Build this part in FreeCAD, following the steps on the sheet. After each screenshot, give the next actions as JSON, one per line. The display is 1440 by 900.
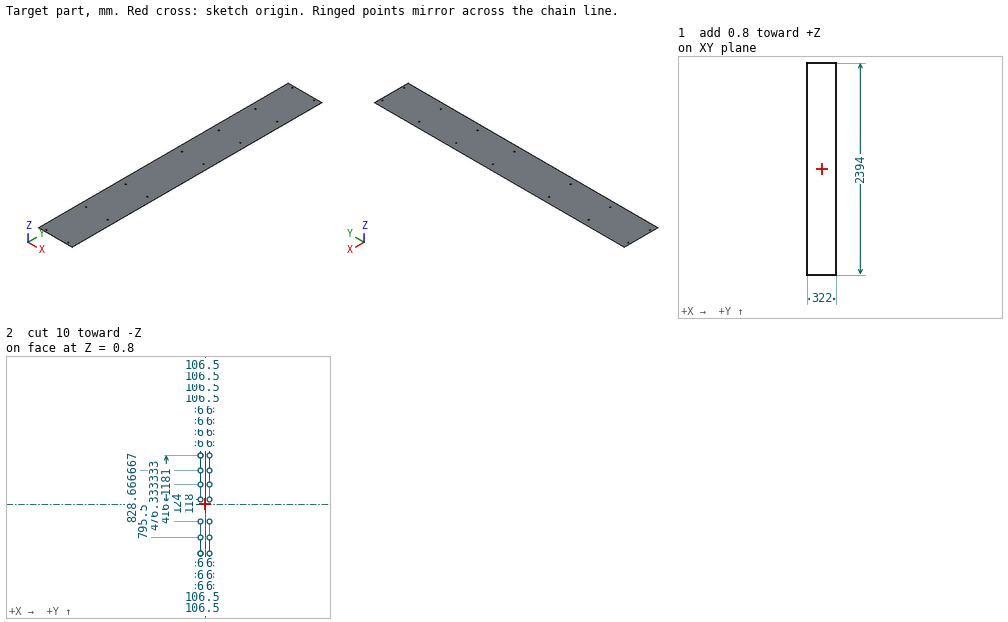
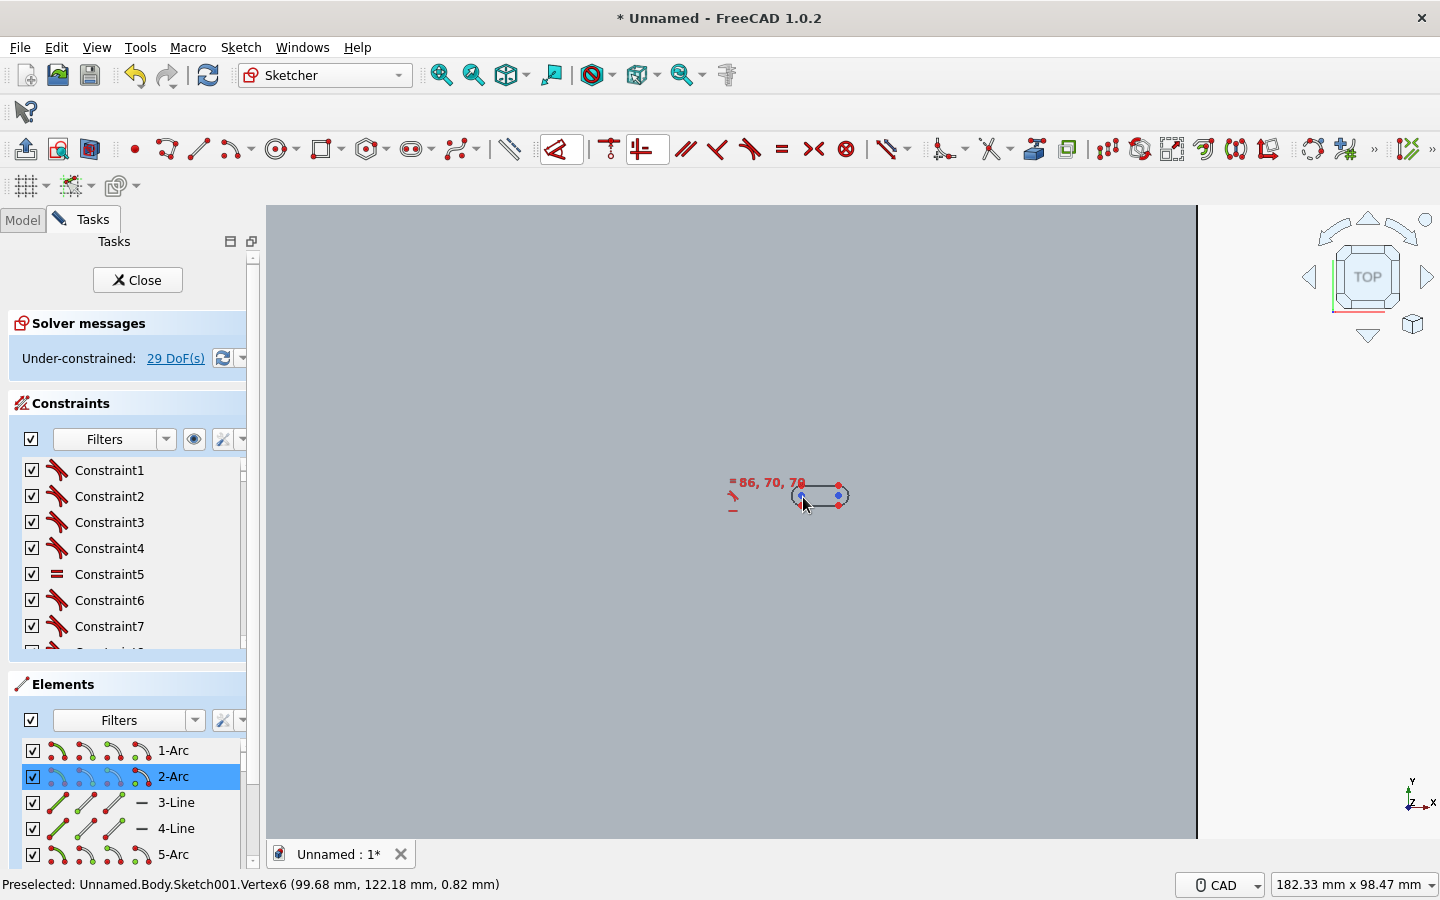
{"action": "scroll", "coordinate": [802, 496], "scroll_direction": "up", "scroll_amount": 4}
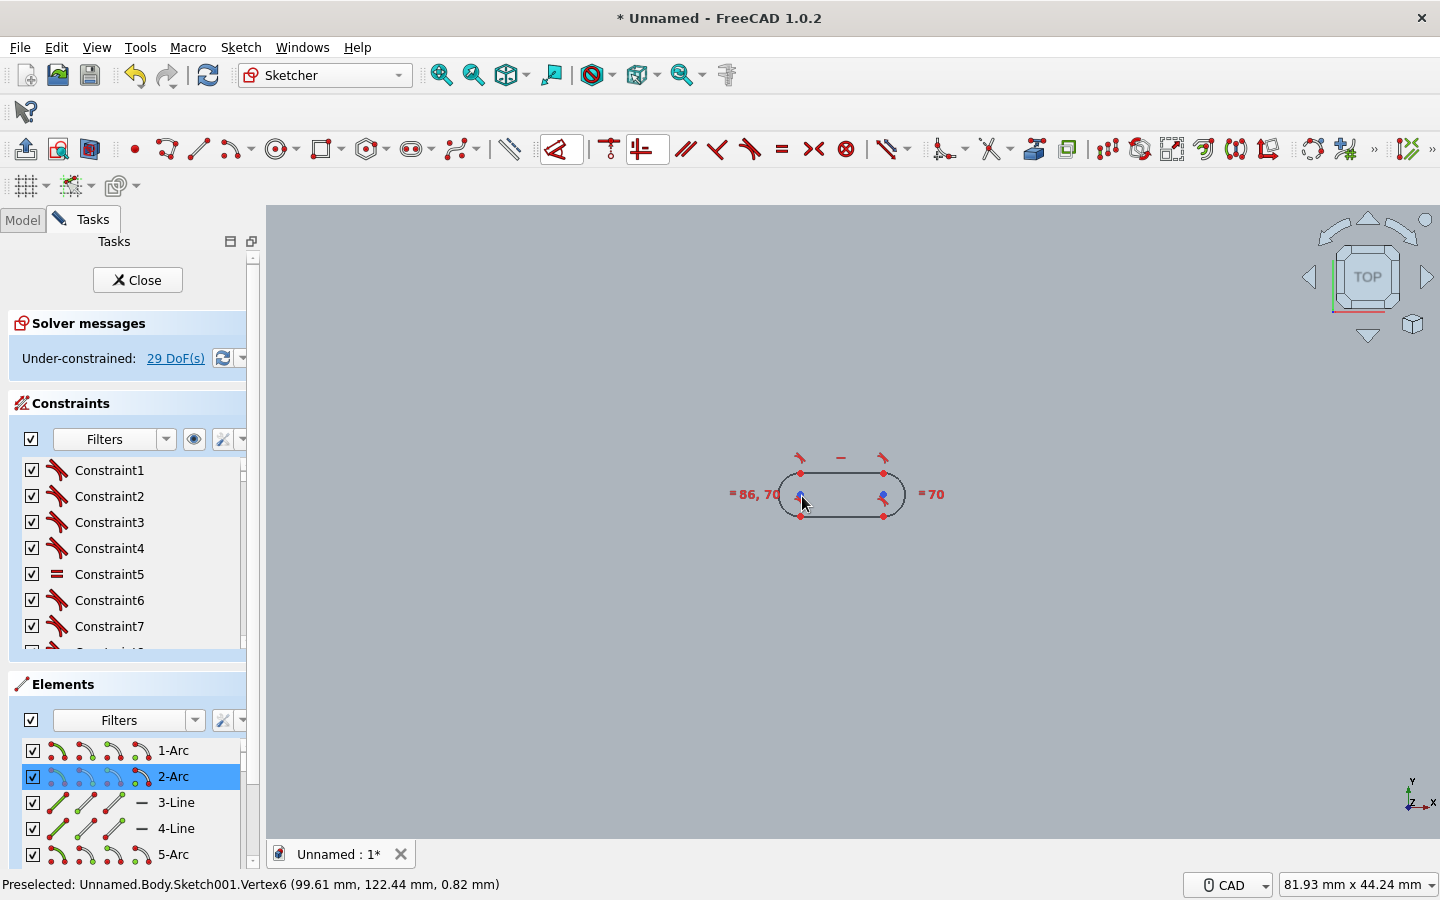
{"action": "left_click", "coordinate": [800, 495]}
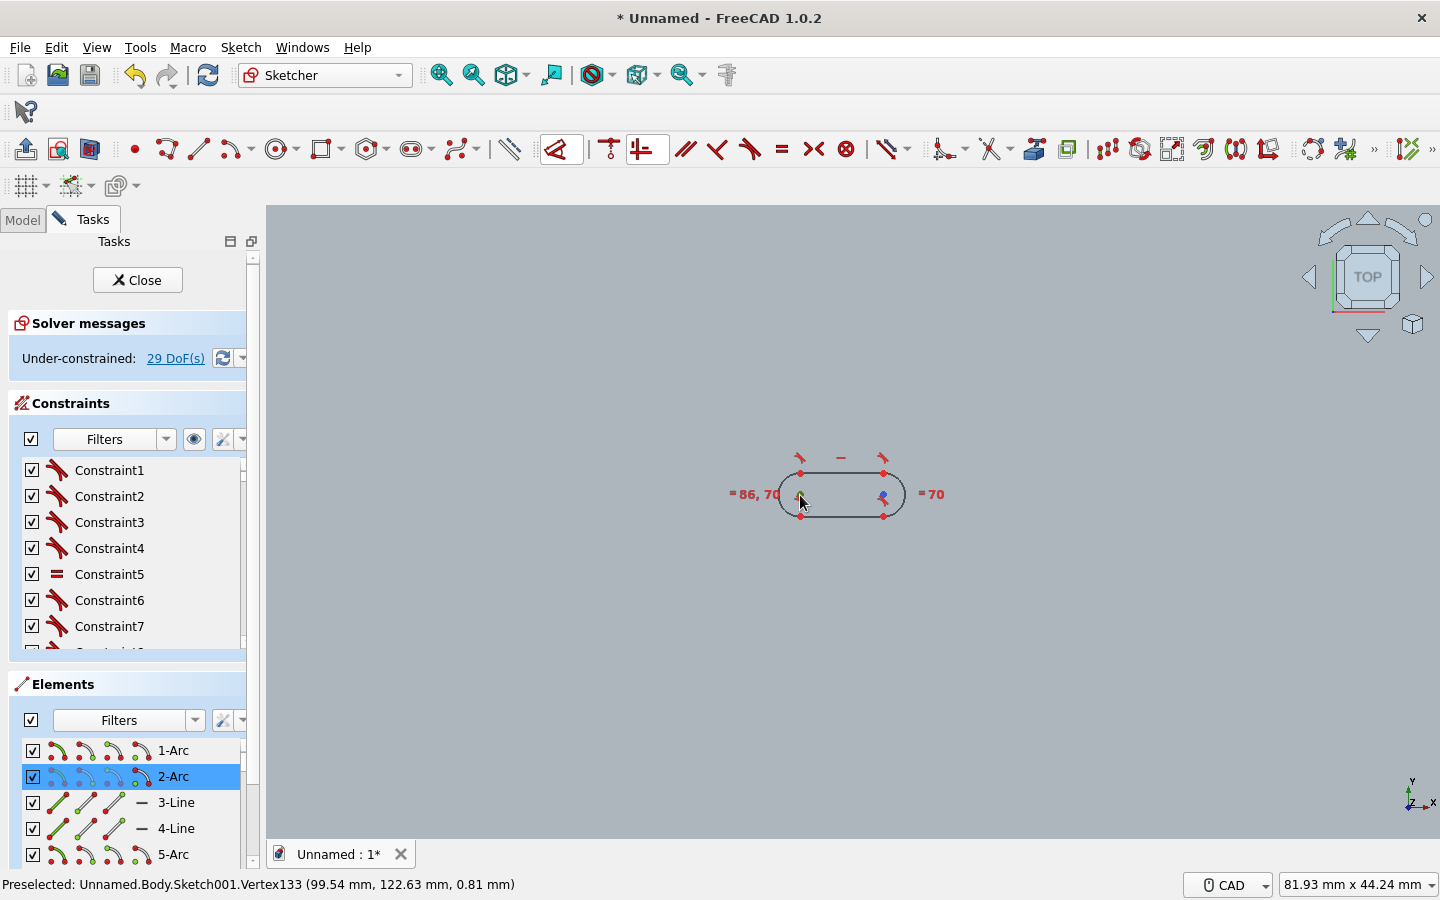
{"action": "scroll", "coordinate": [784, 522], "scroll_direction": "down", "scroll_amount": 15}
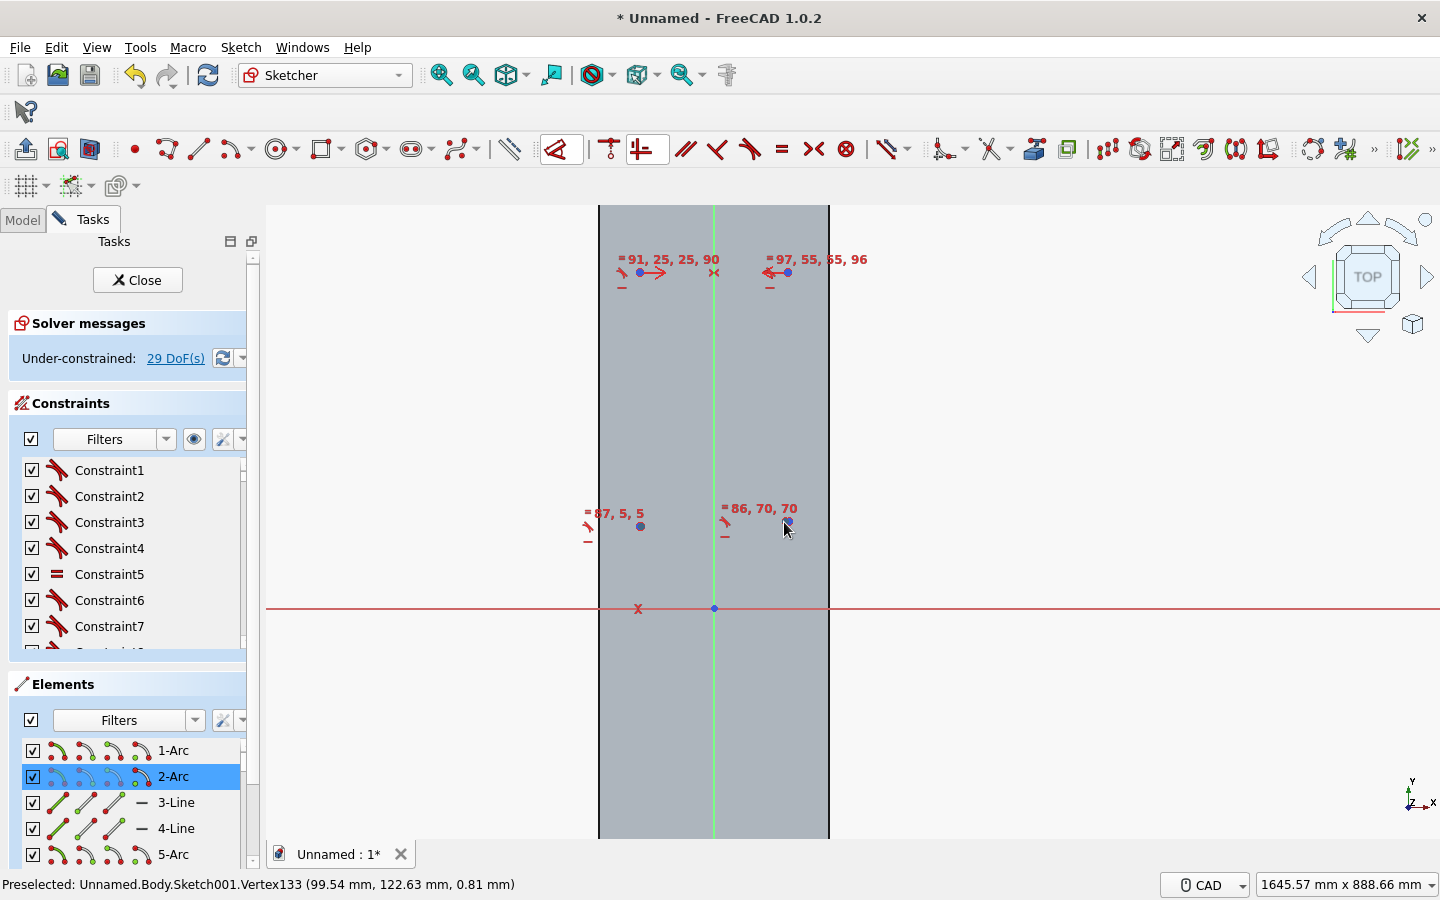
{"action": "scroll", "coordinate": [808, 494], "scroll_direction": "down", "scroll_amount": 7}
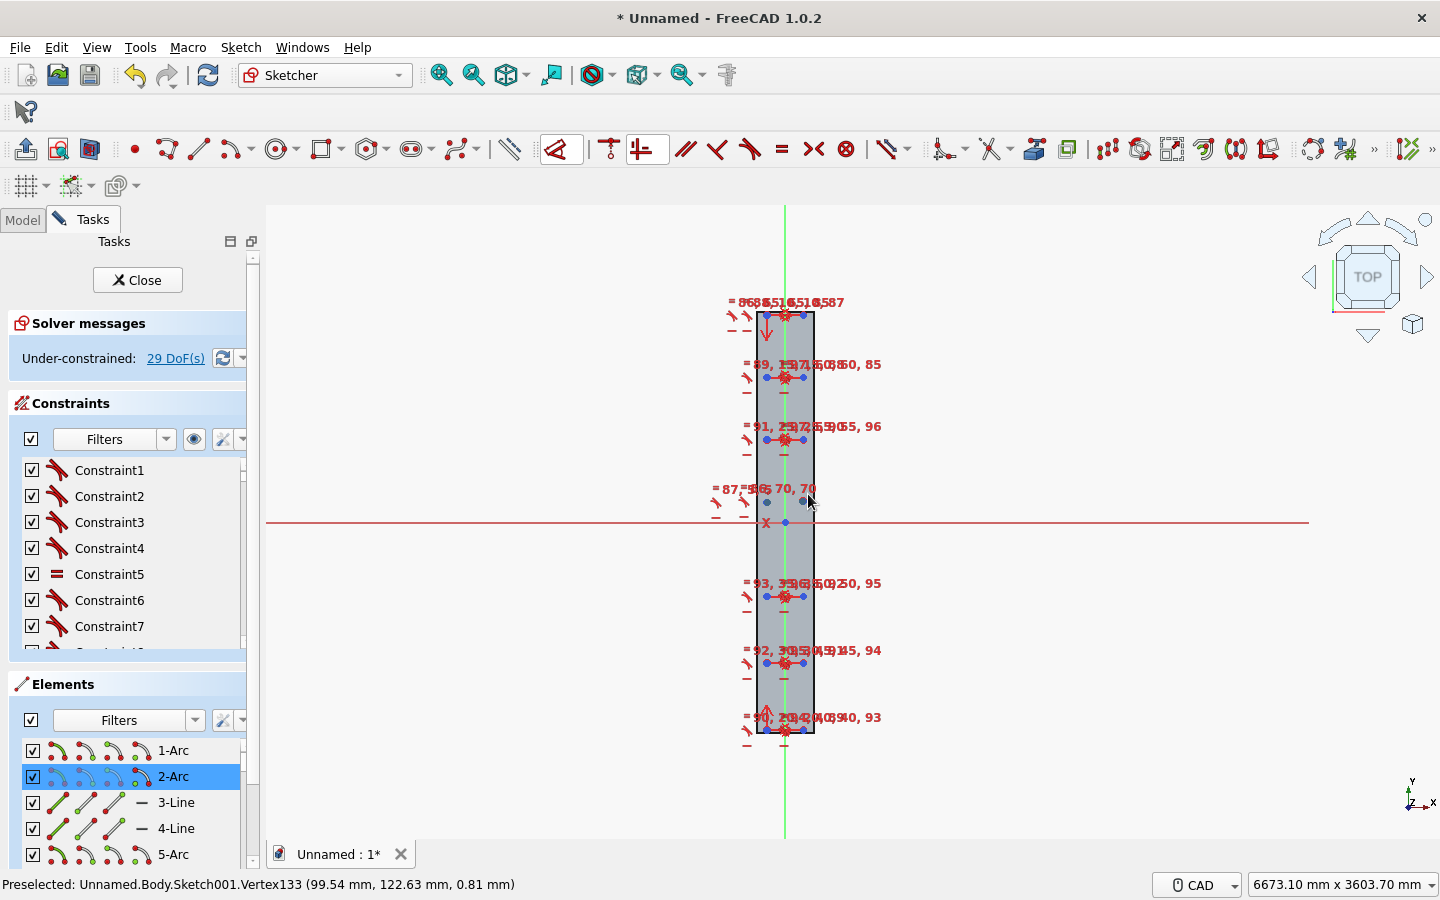
{"action": "left_click", "coordinate": [785, 770]}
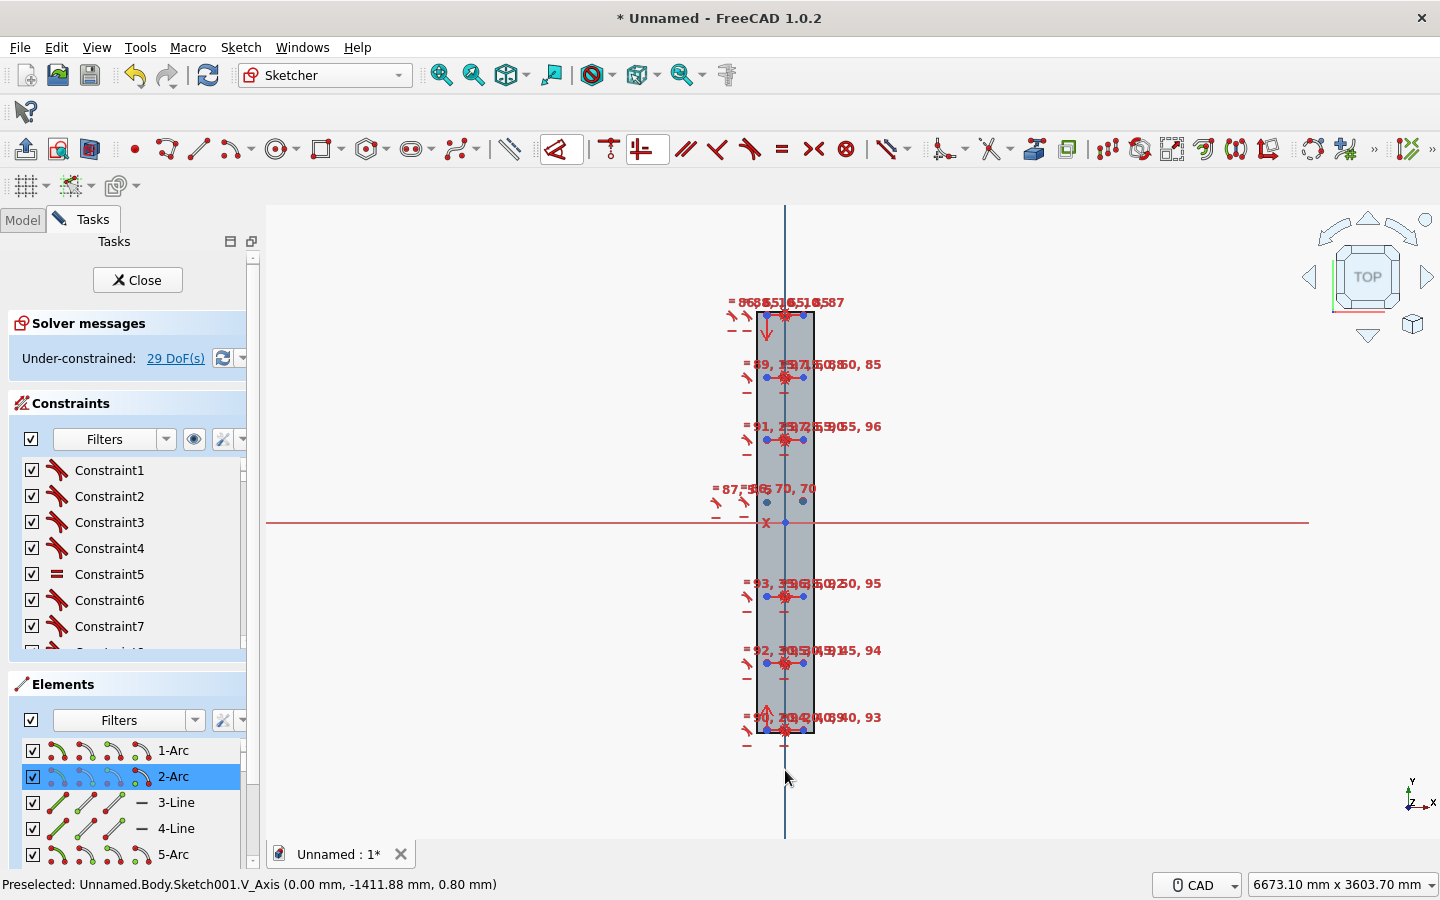
{"action": "left_click", "coordinate": [814, 150]}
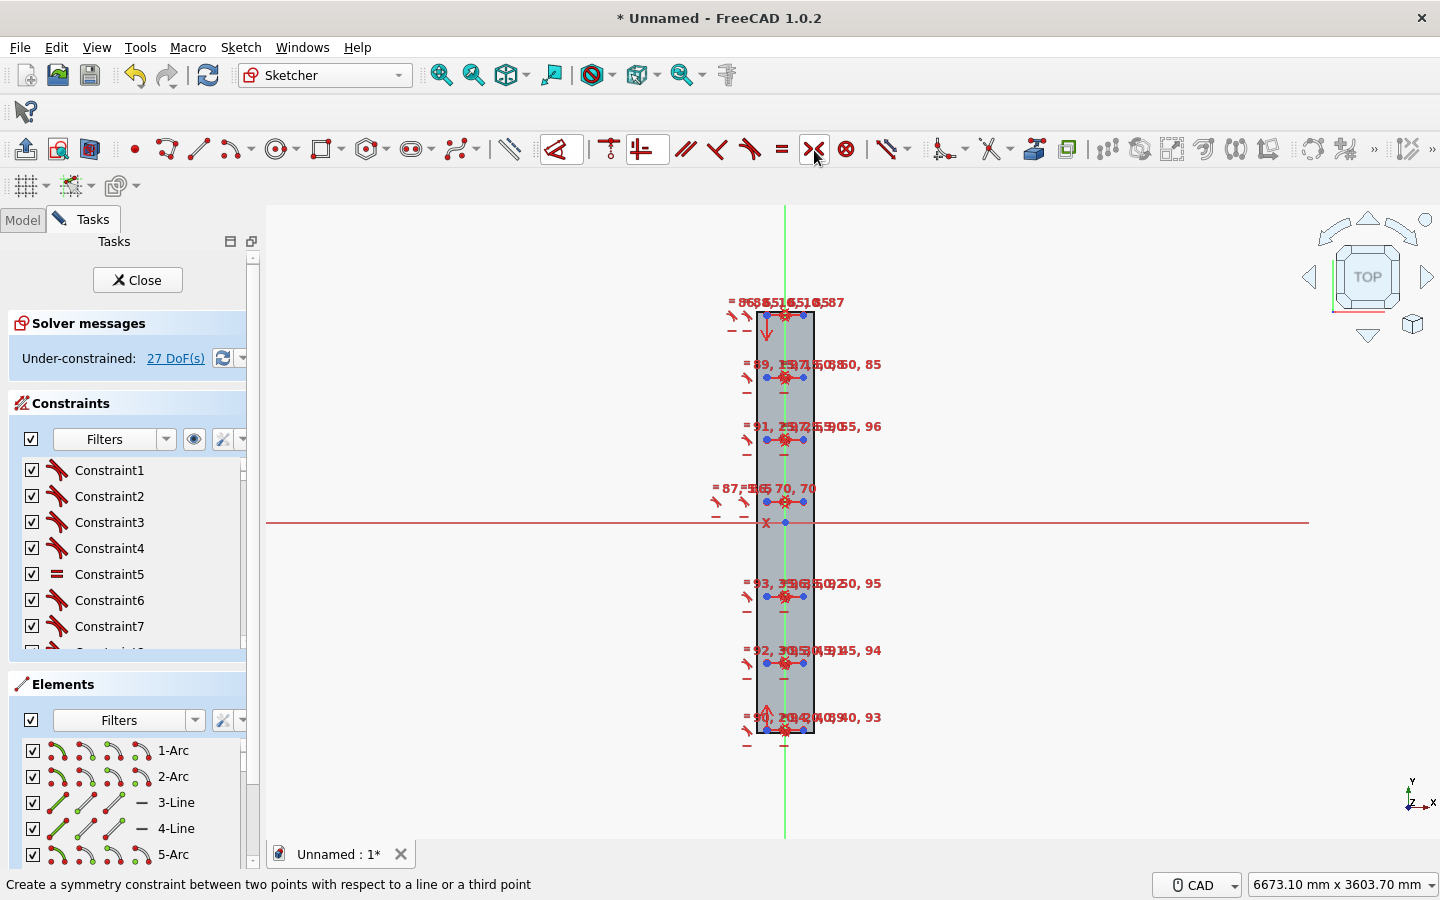
{"action": "scroll", "coordinate": [767, 502], "scroll_direction": "up", "scroll_amount": 19}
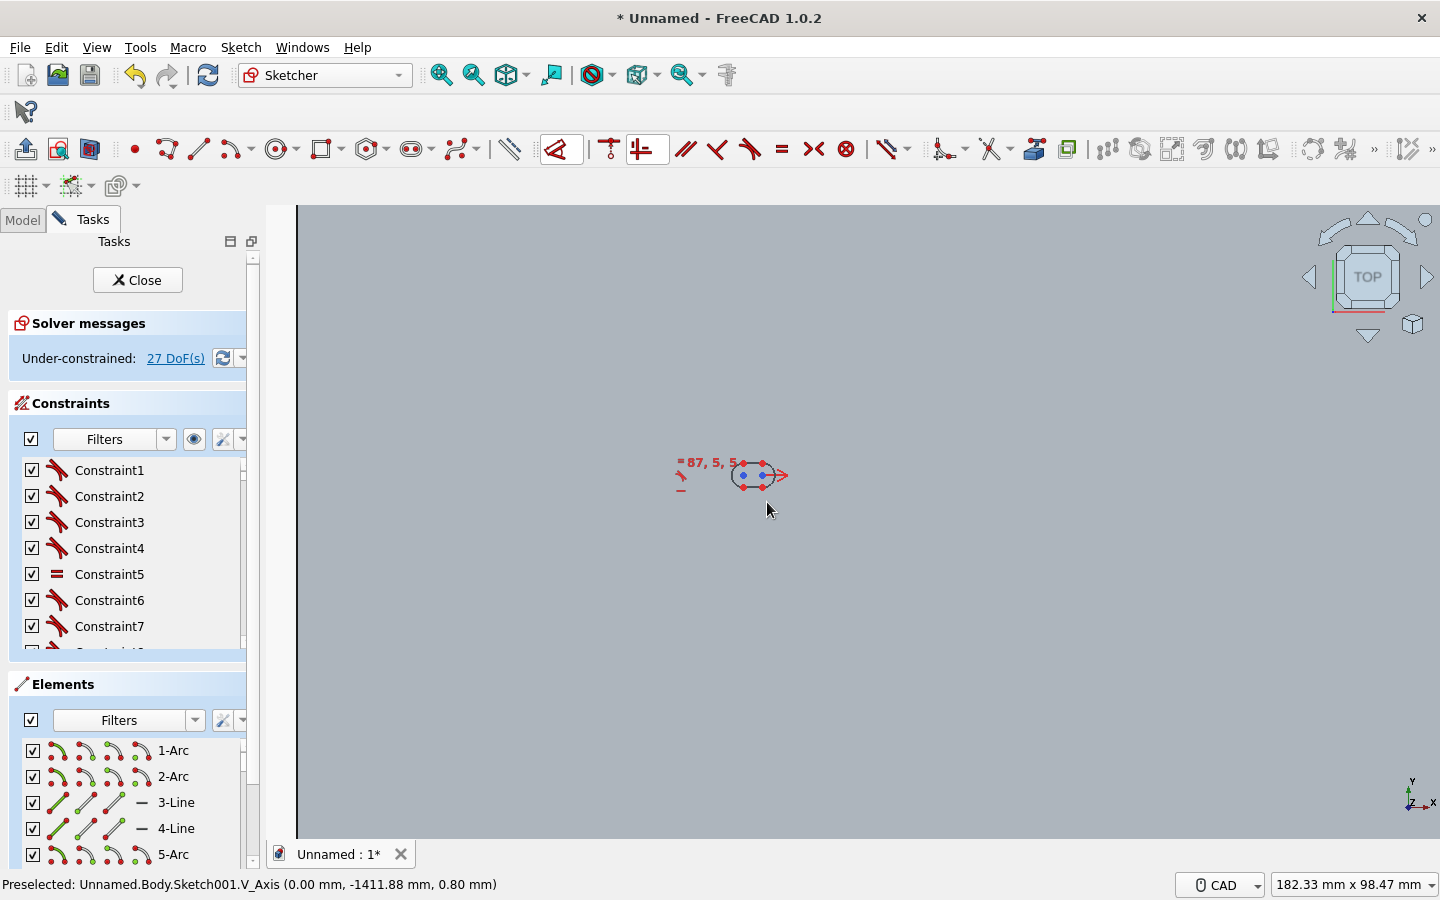
{"action": "left_click", "coordinate": [753, 463]}